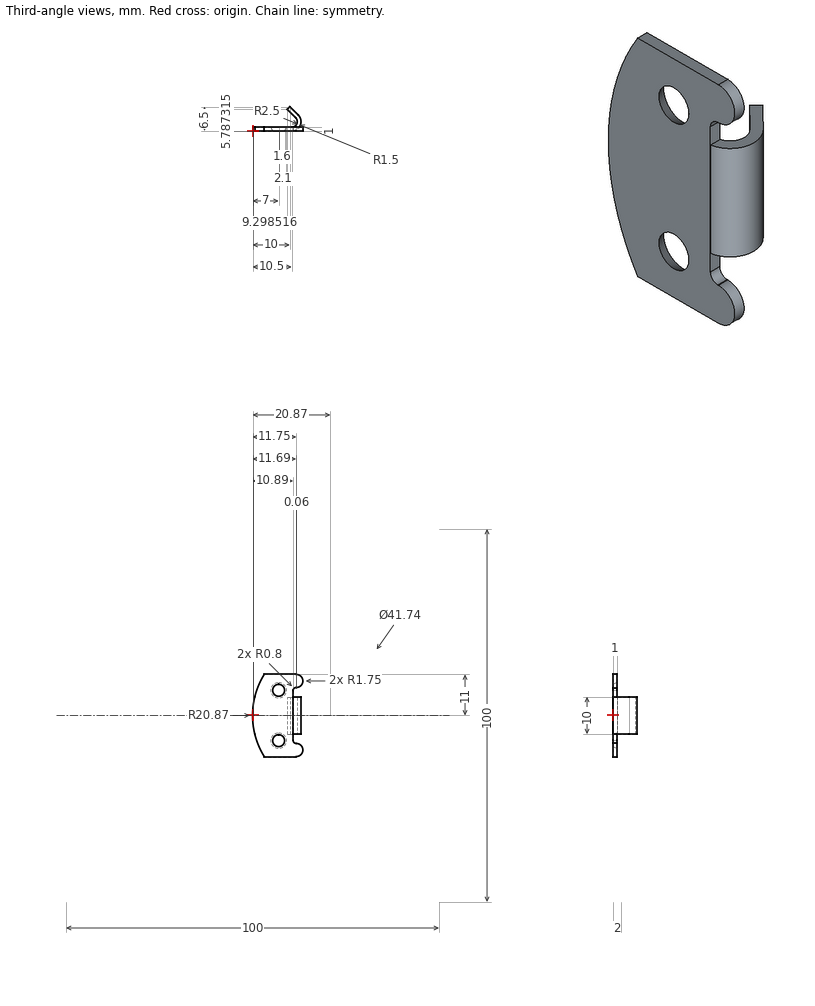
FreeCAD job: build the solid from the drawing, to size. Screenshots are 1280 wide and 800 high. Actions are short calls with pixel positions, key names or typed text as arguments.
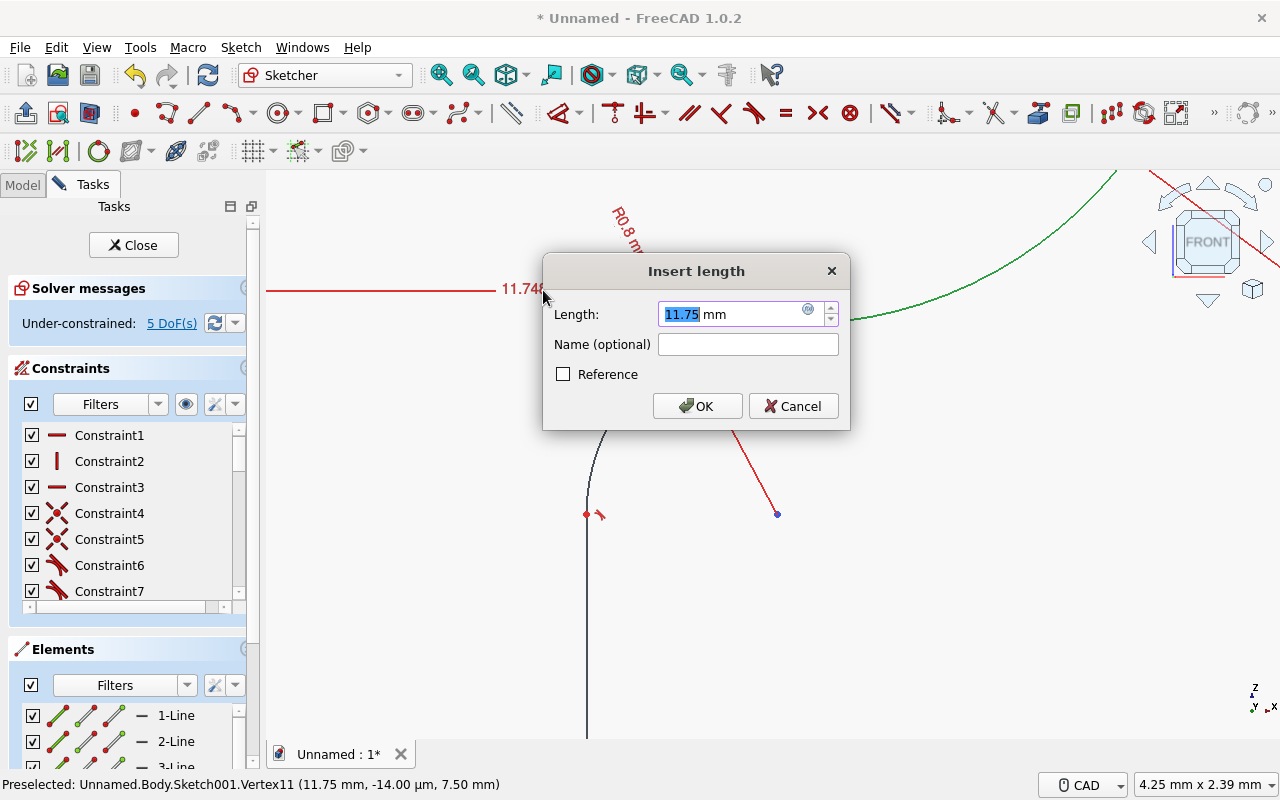
text(11.75)
key(Return)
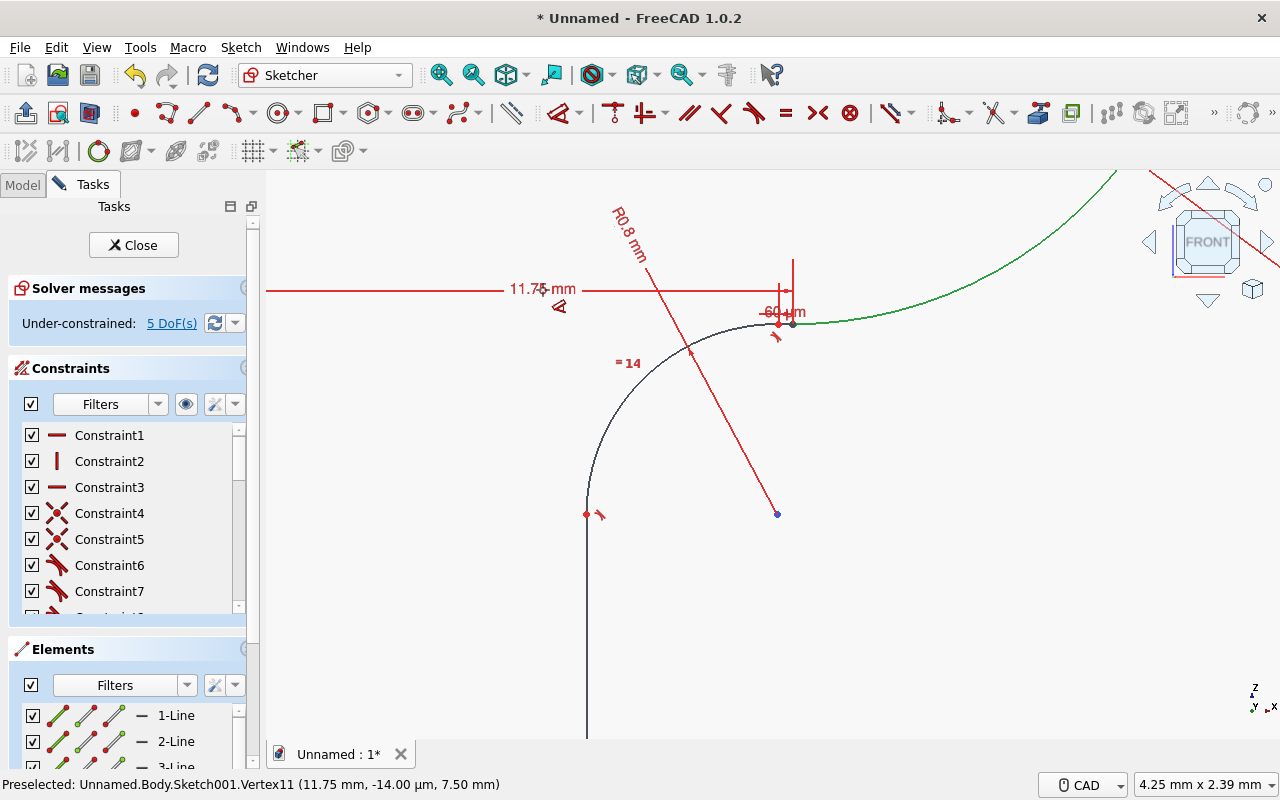
click(779, 324)
click(425, 290)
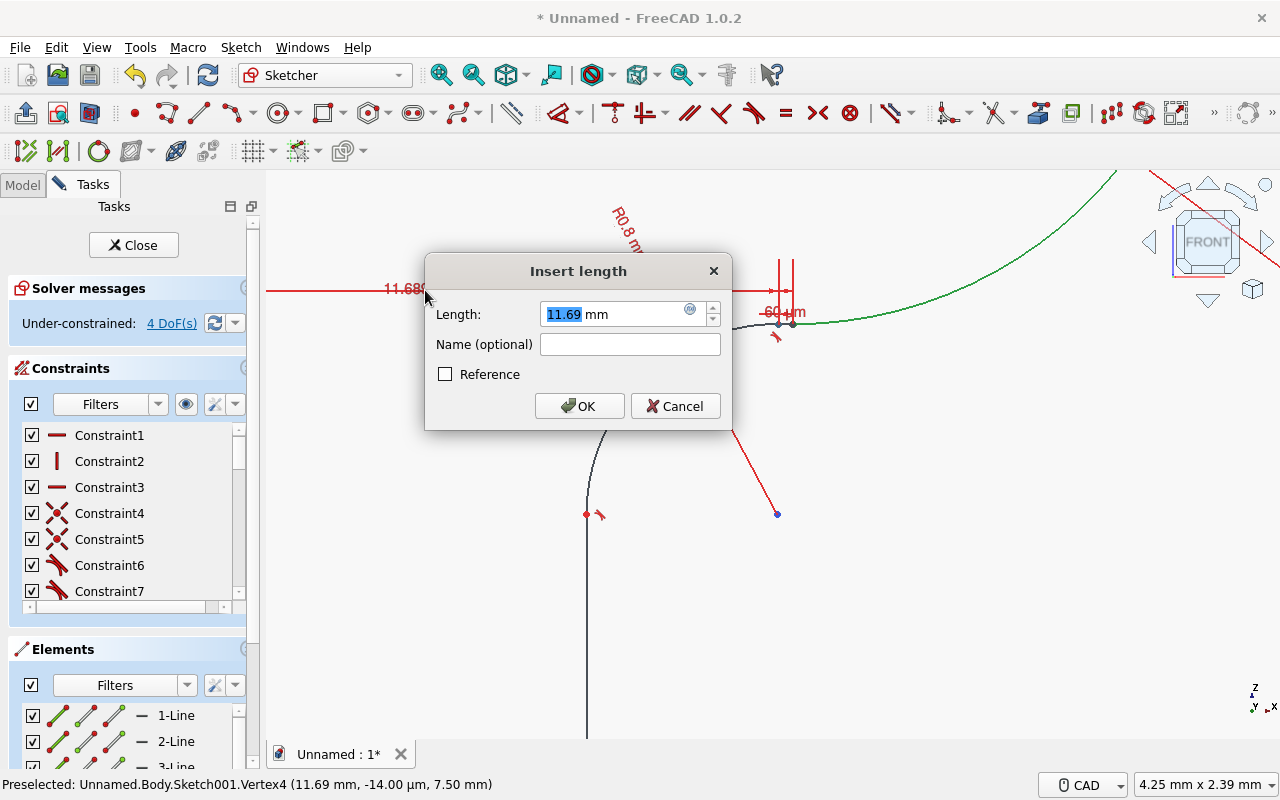
text(11.69)
key(Return)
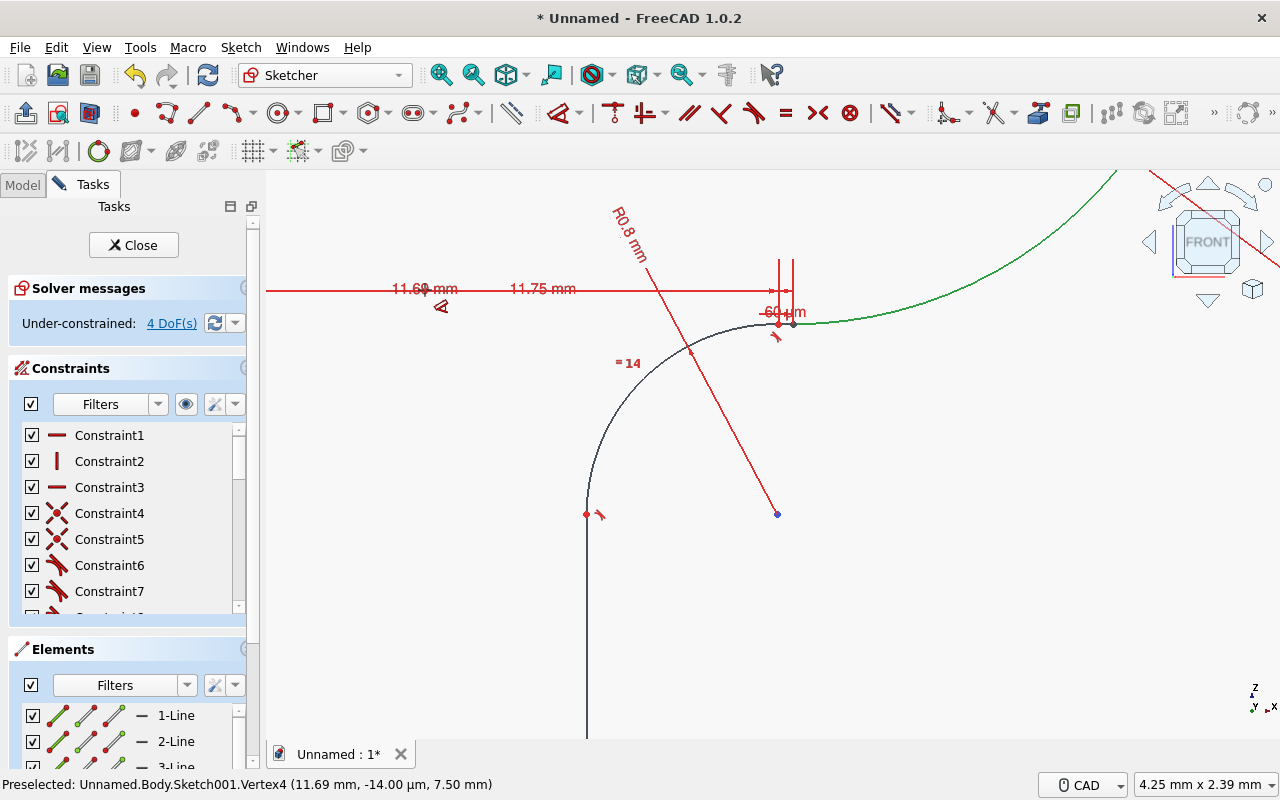
scroll(793, 322, down, 13)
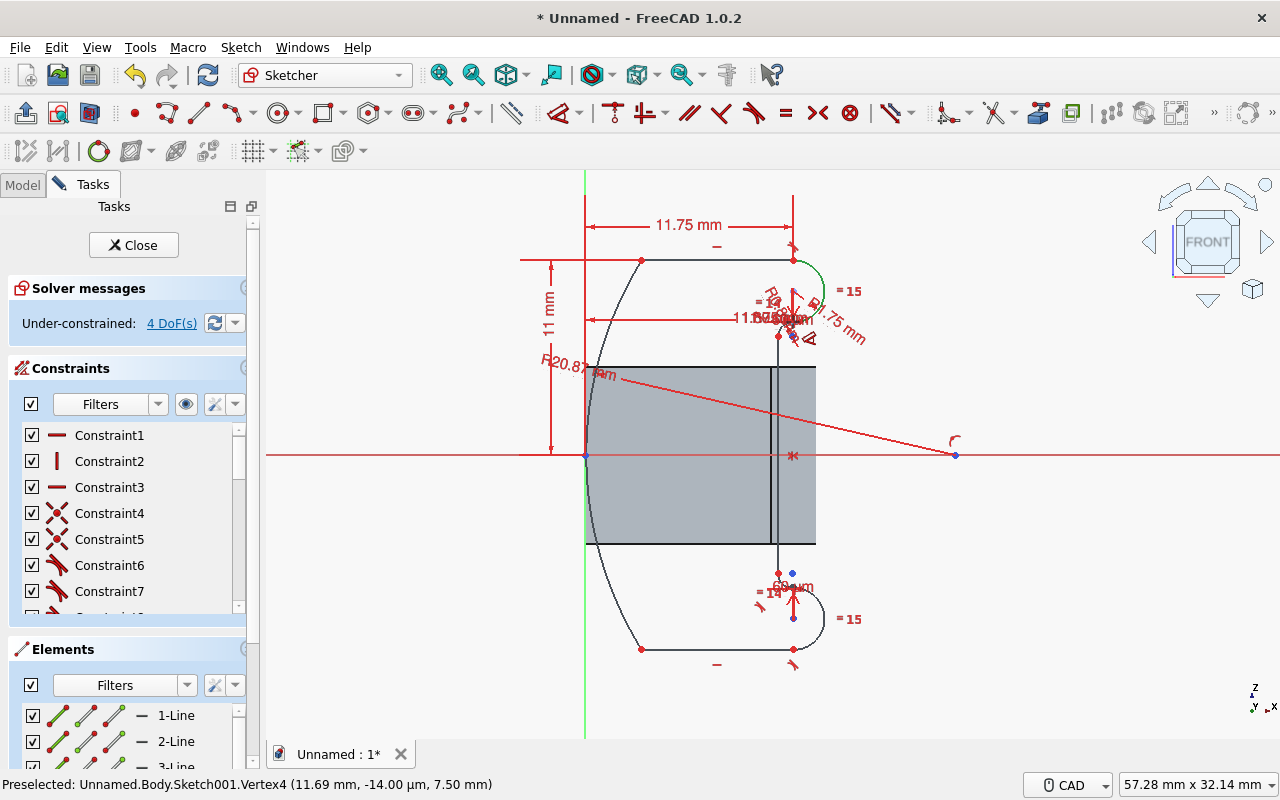
click(778, 337)
click(682, 303)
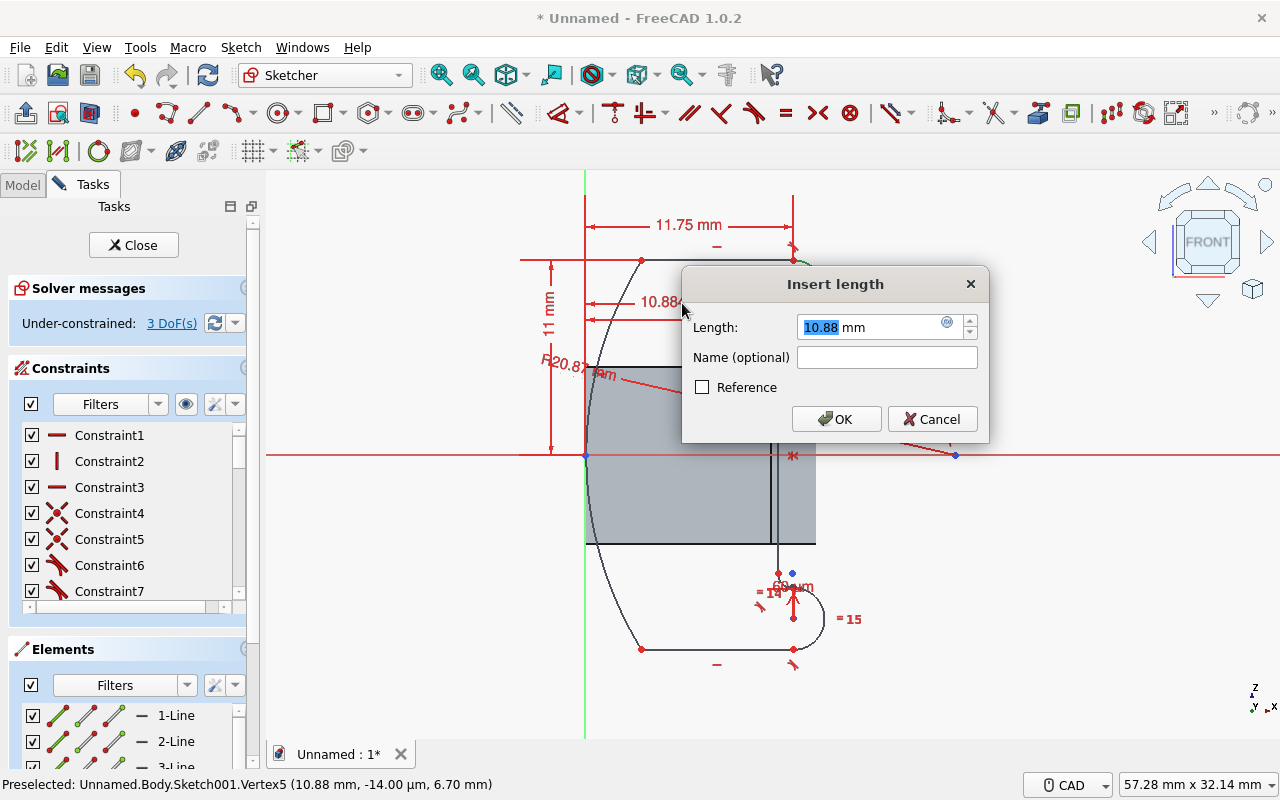
text(10.89)
key(Return)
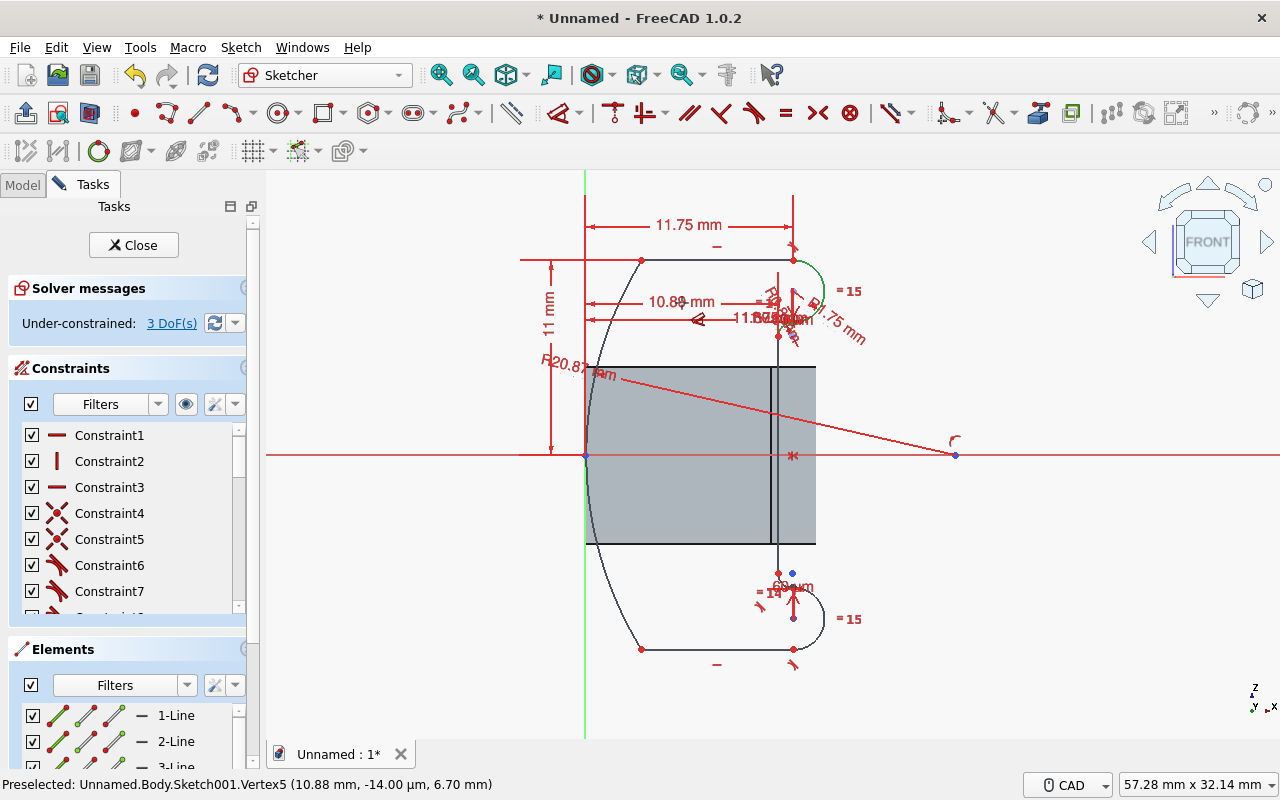
scroll(793, 588, up, 13)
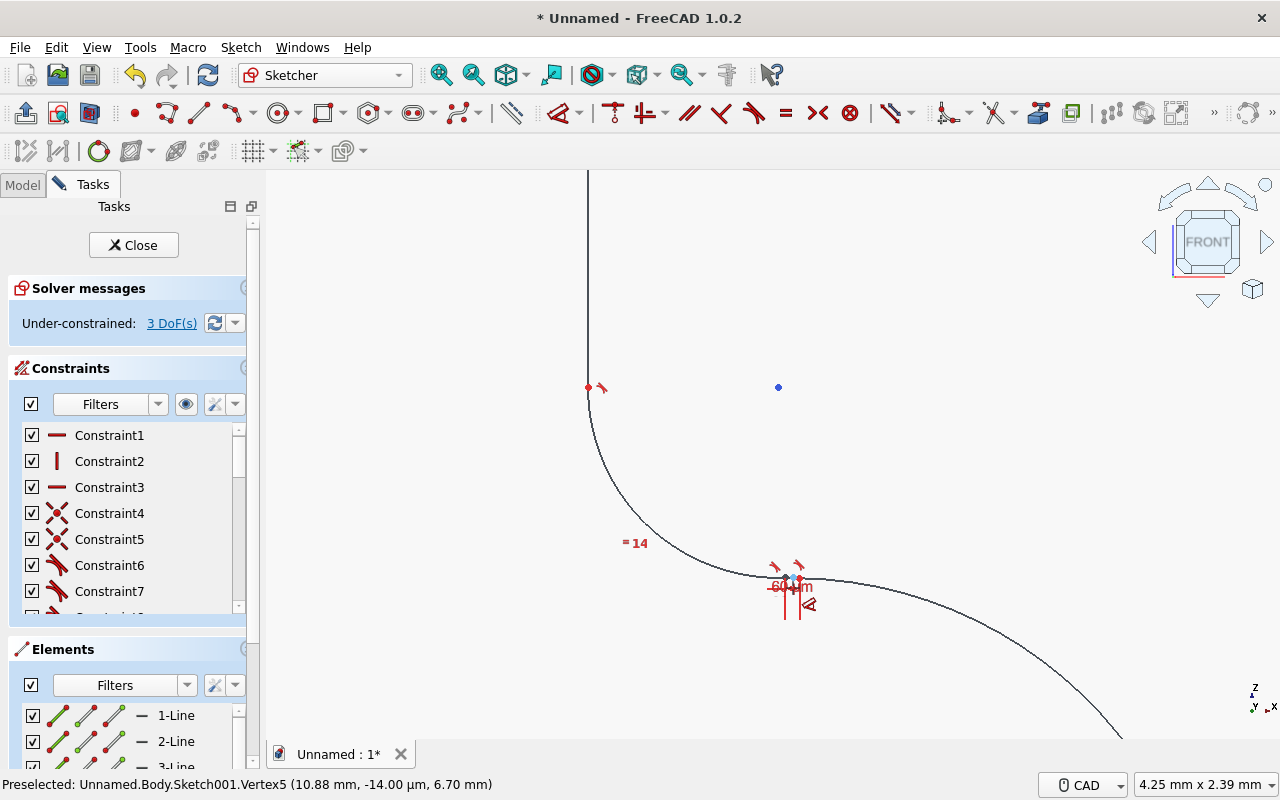
click(785, 578)
click(540, 612)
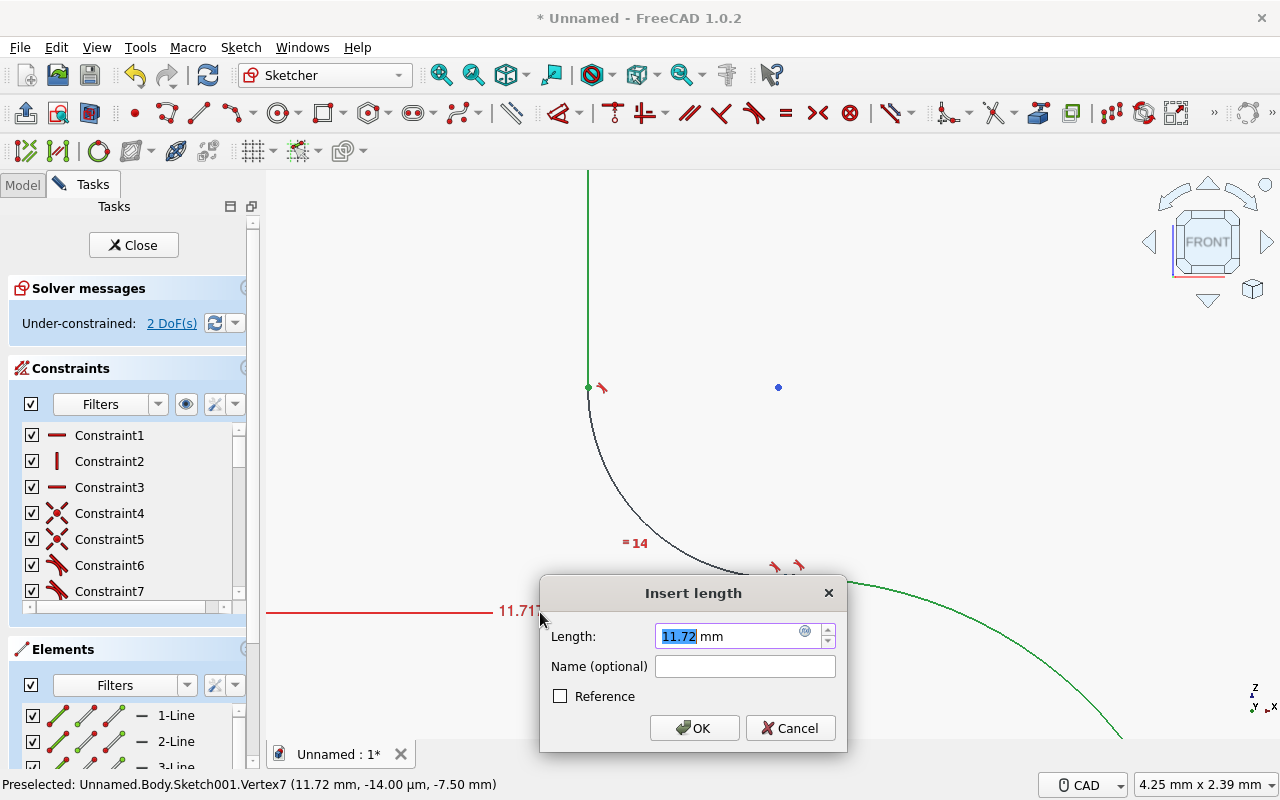
text(11.69)
key(Return)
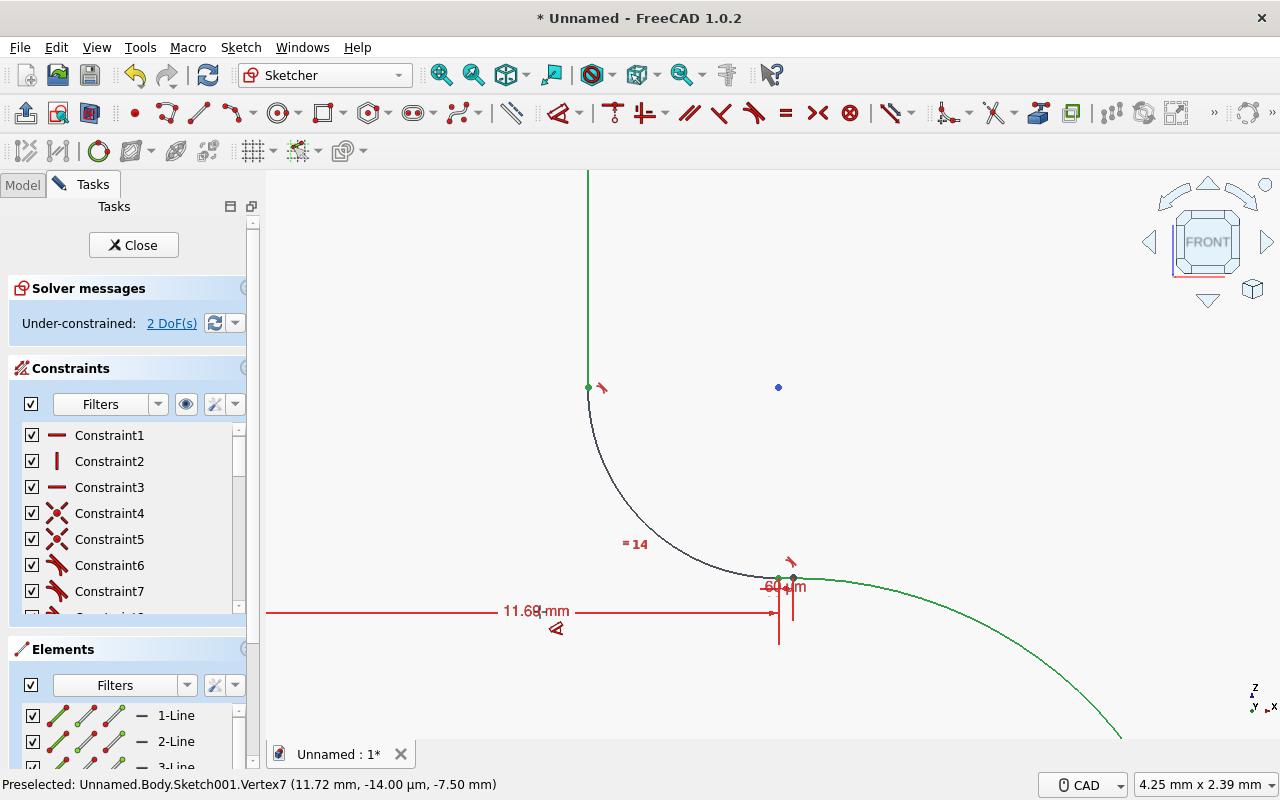
click(794, 578)
click(429, 612)